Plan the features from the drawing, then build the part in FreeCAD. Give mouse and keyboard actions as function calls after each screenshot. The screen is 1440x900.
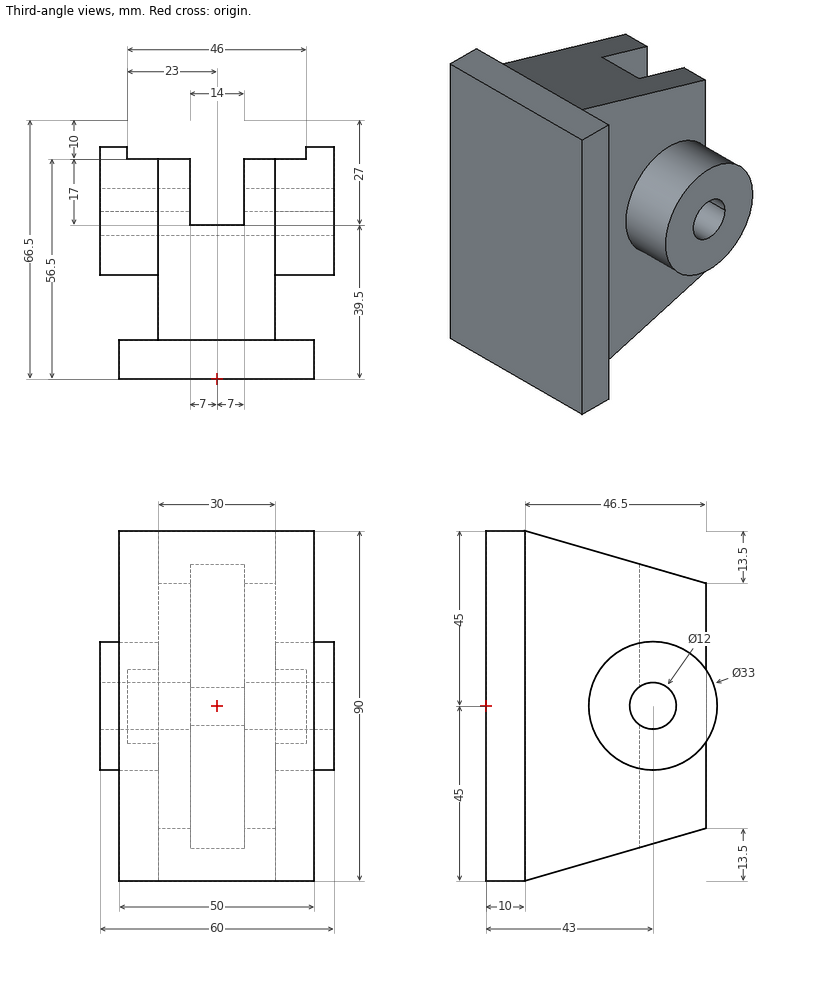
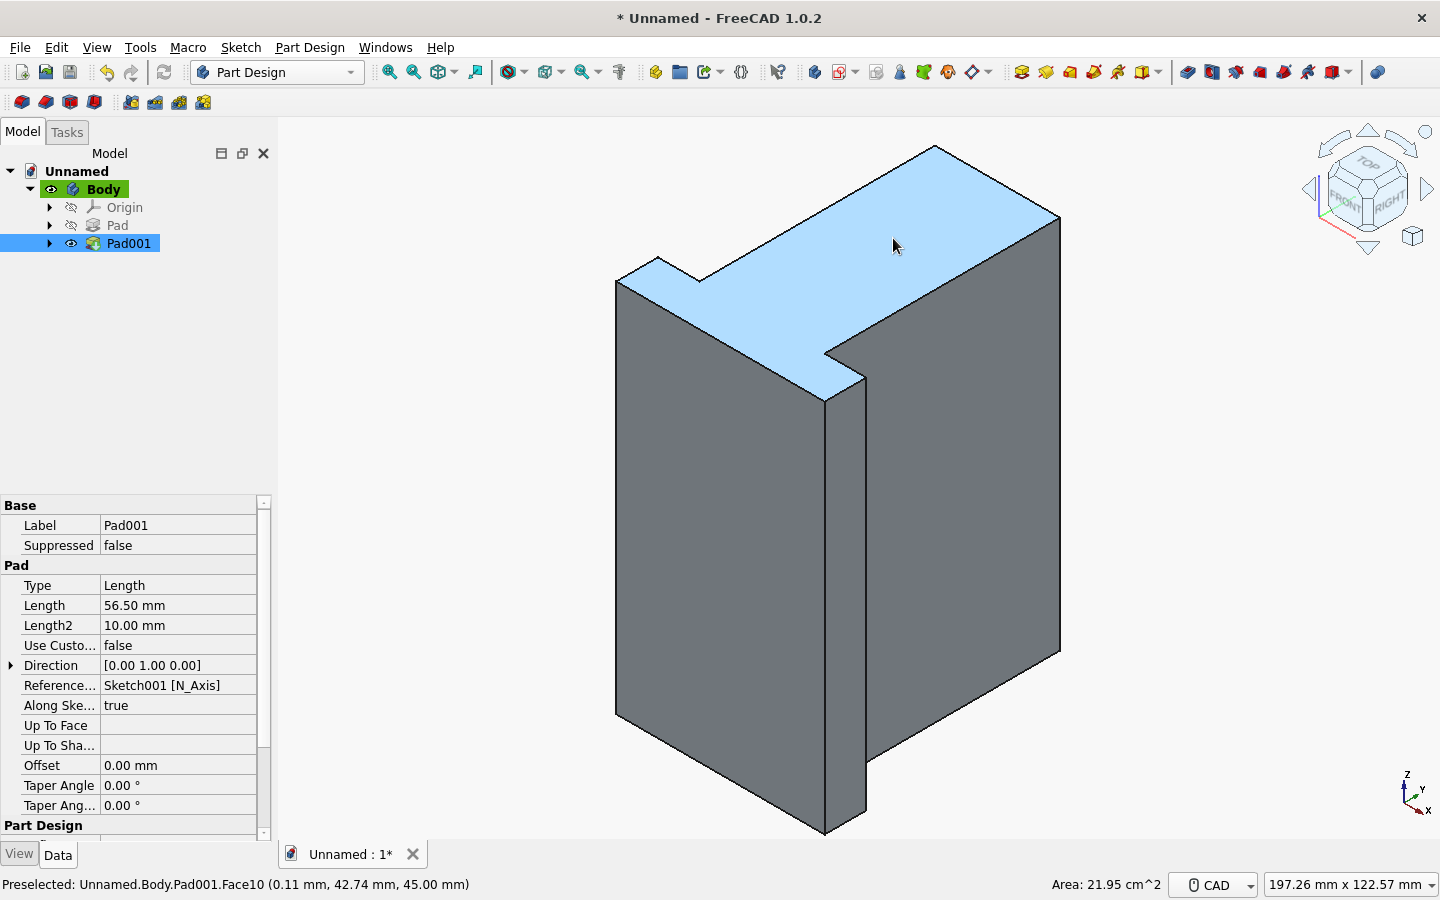
click(840, 72)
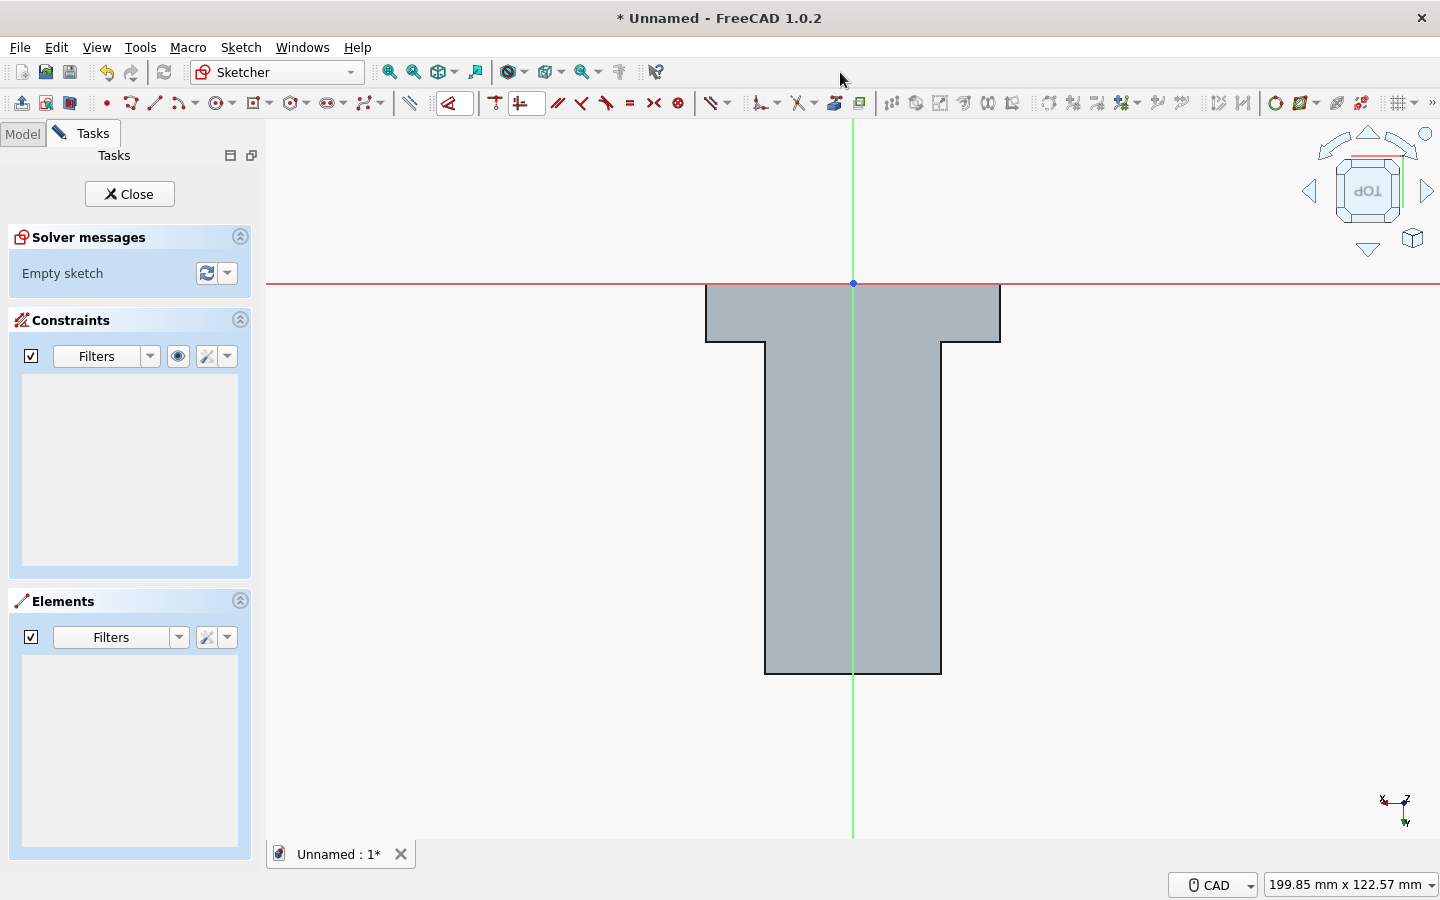
click(272, 104)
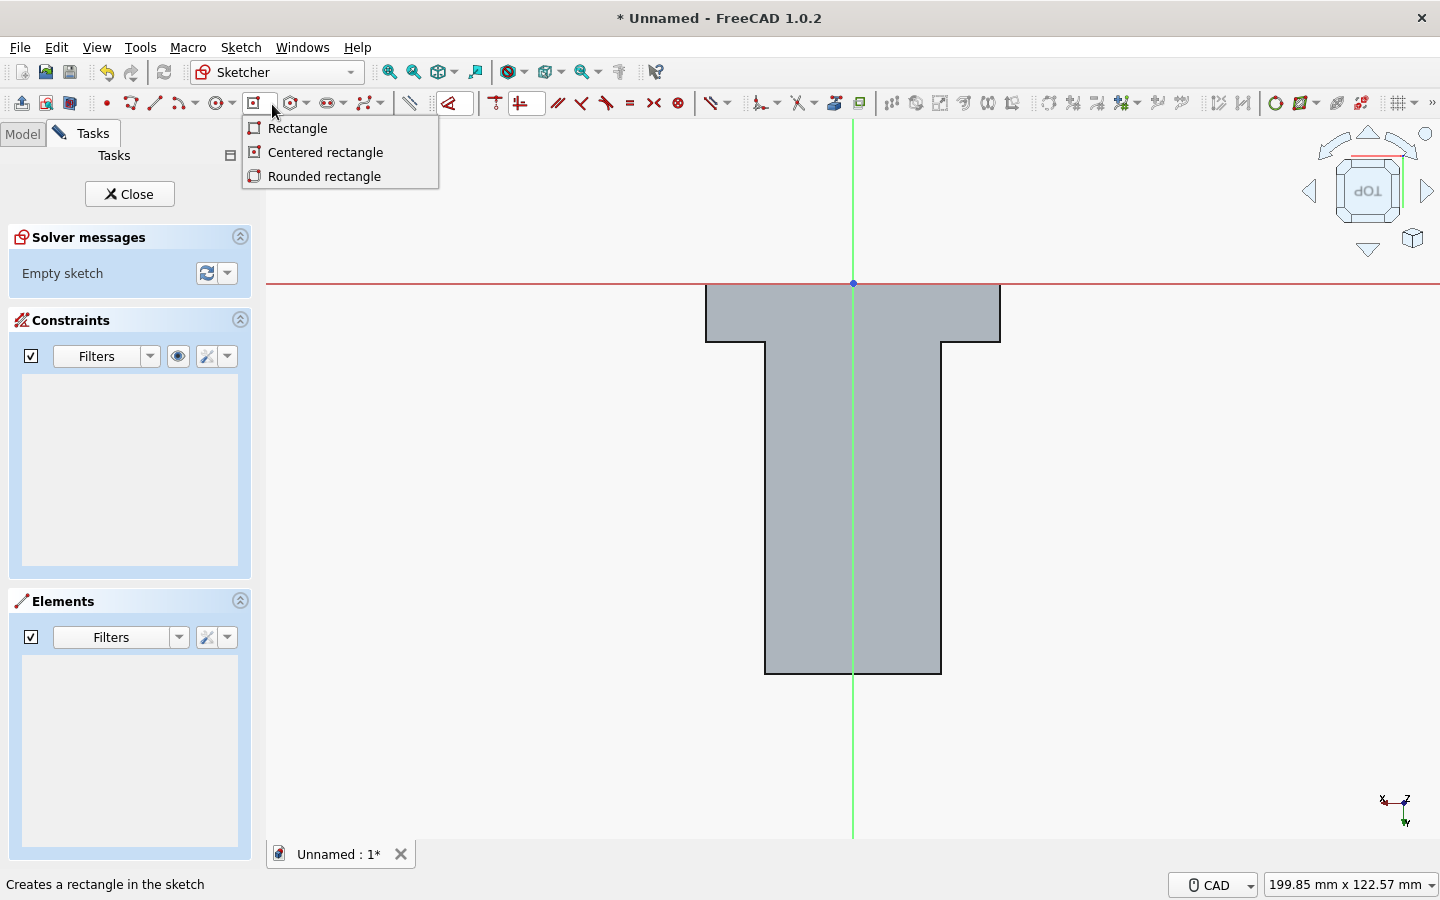
click(340, 128)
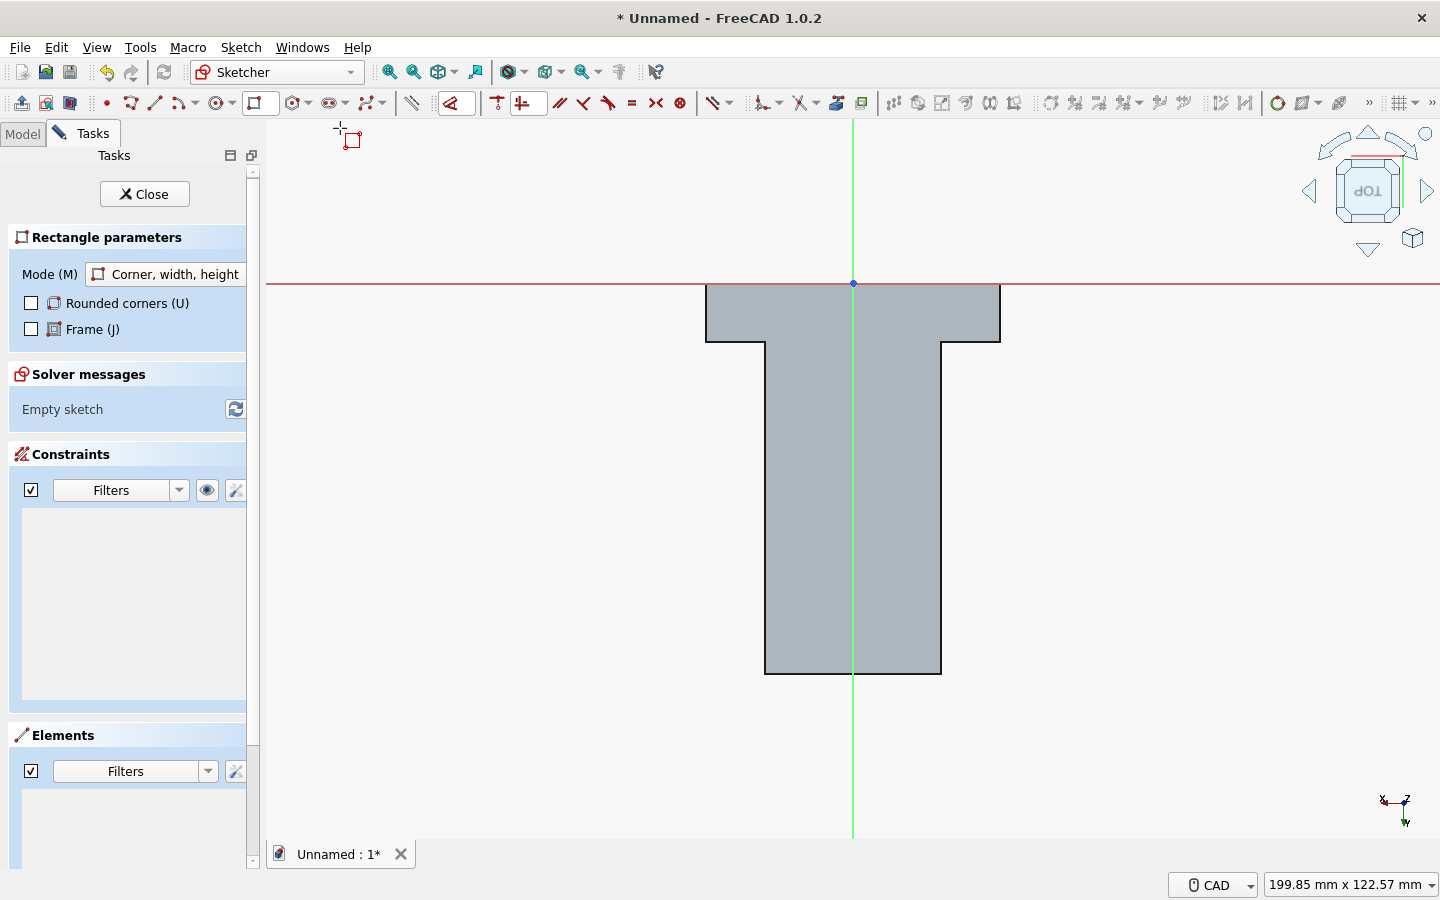
click(812, 516)
click(894, 674)
key(Escape)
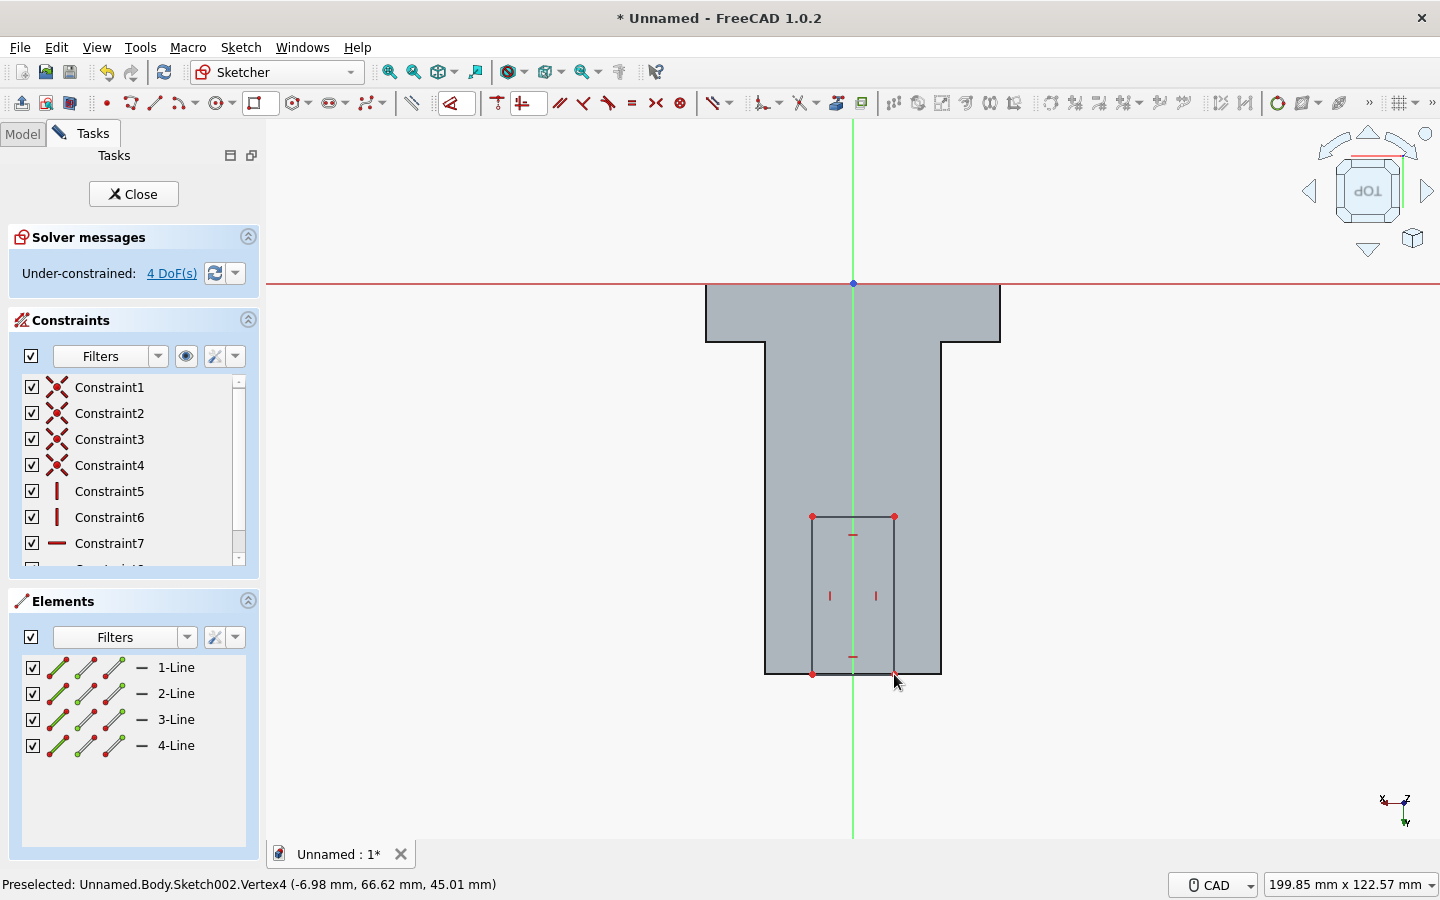
click(812, 564)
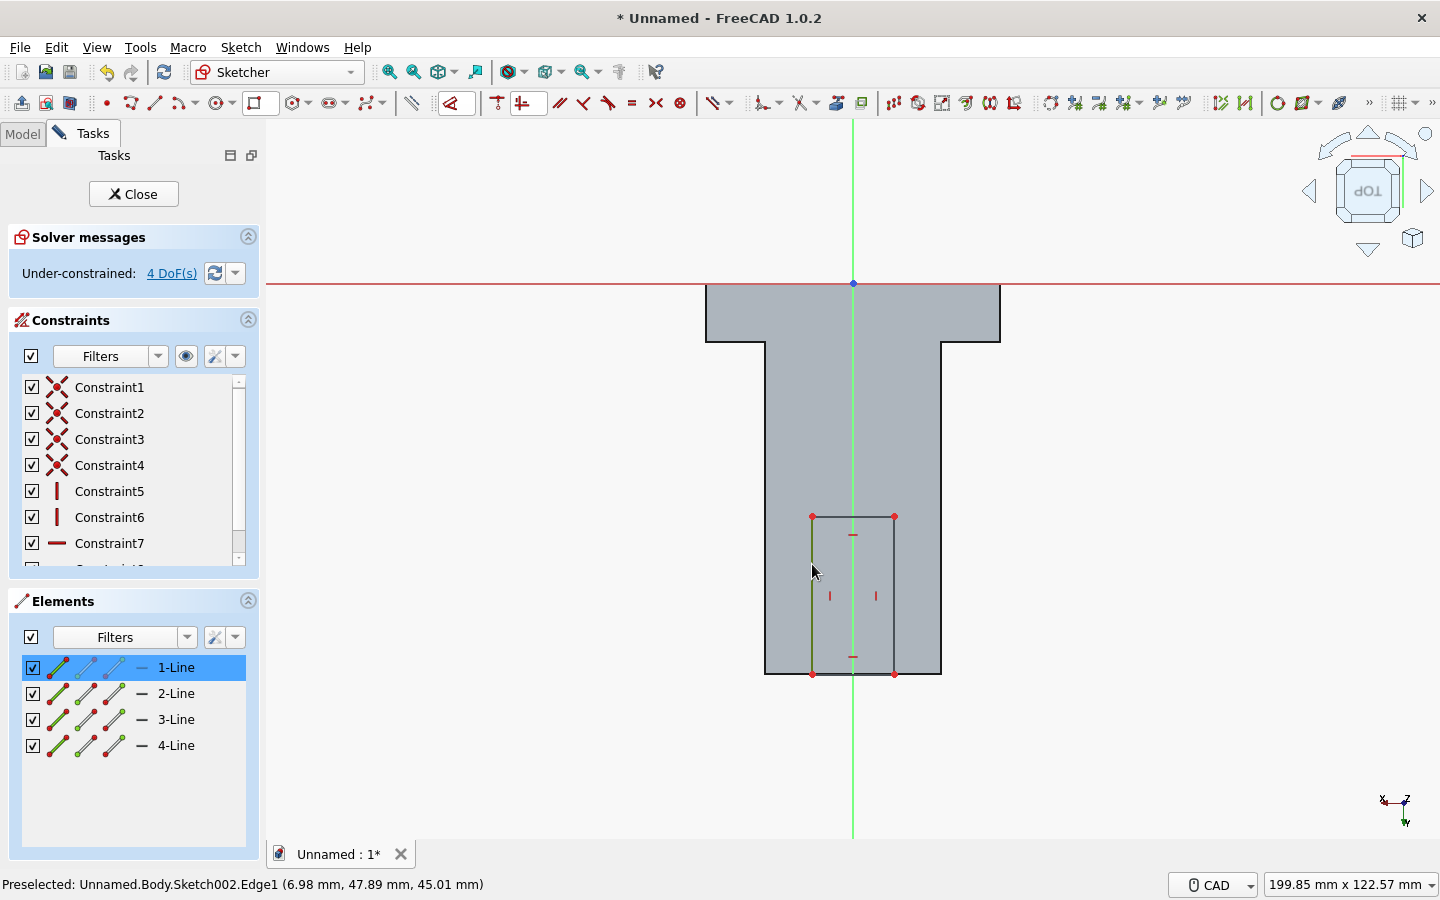
click(470, 104)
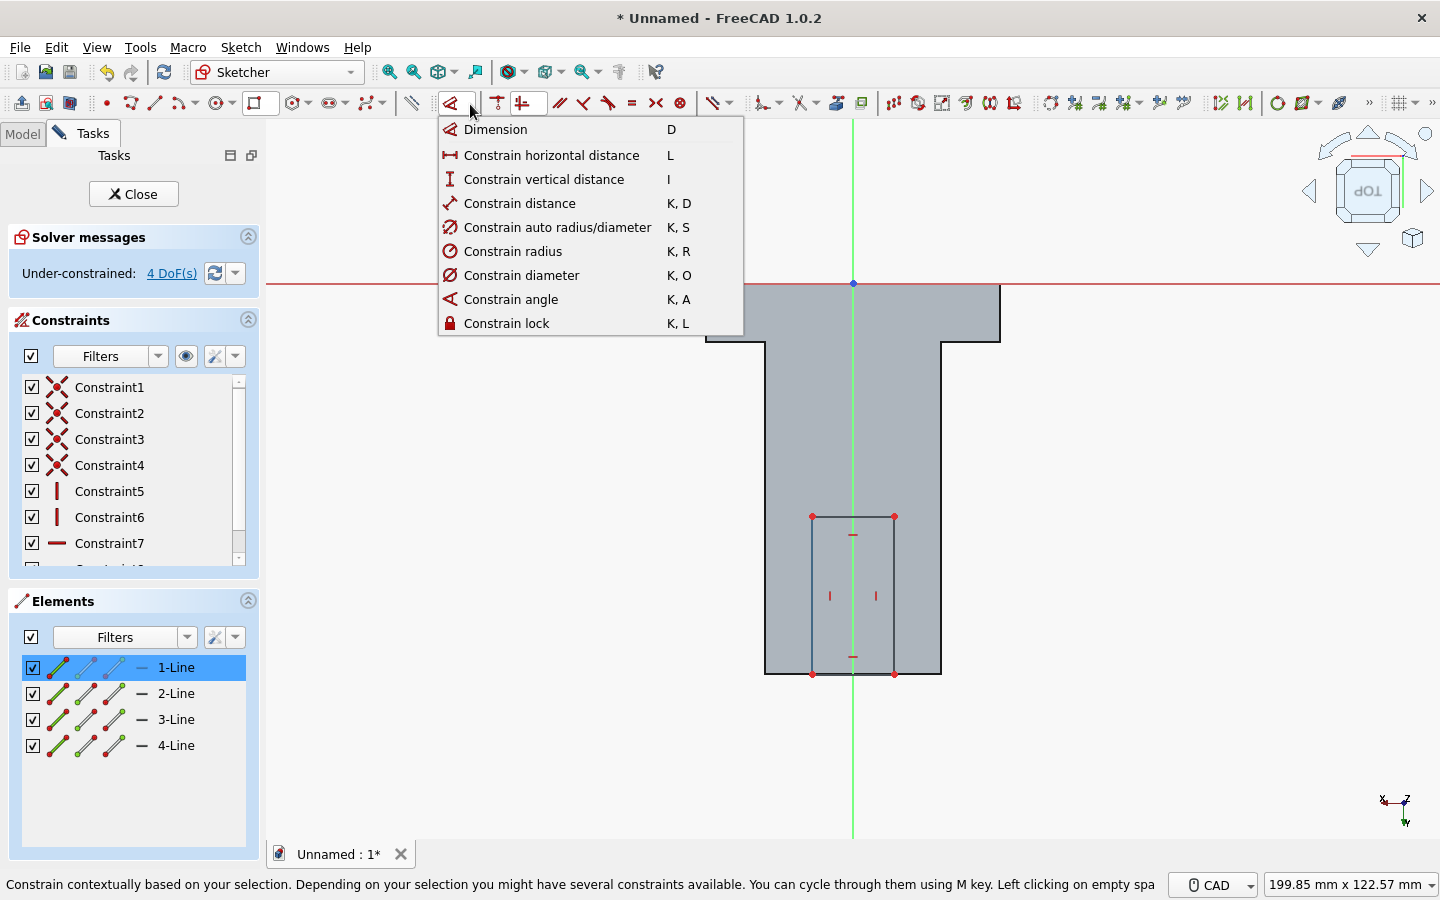
click(591, 179)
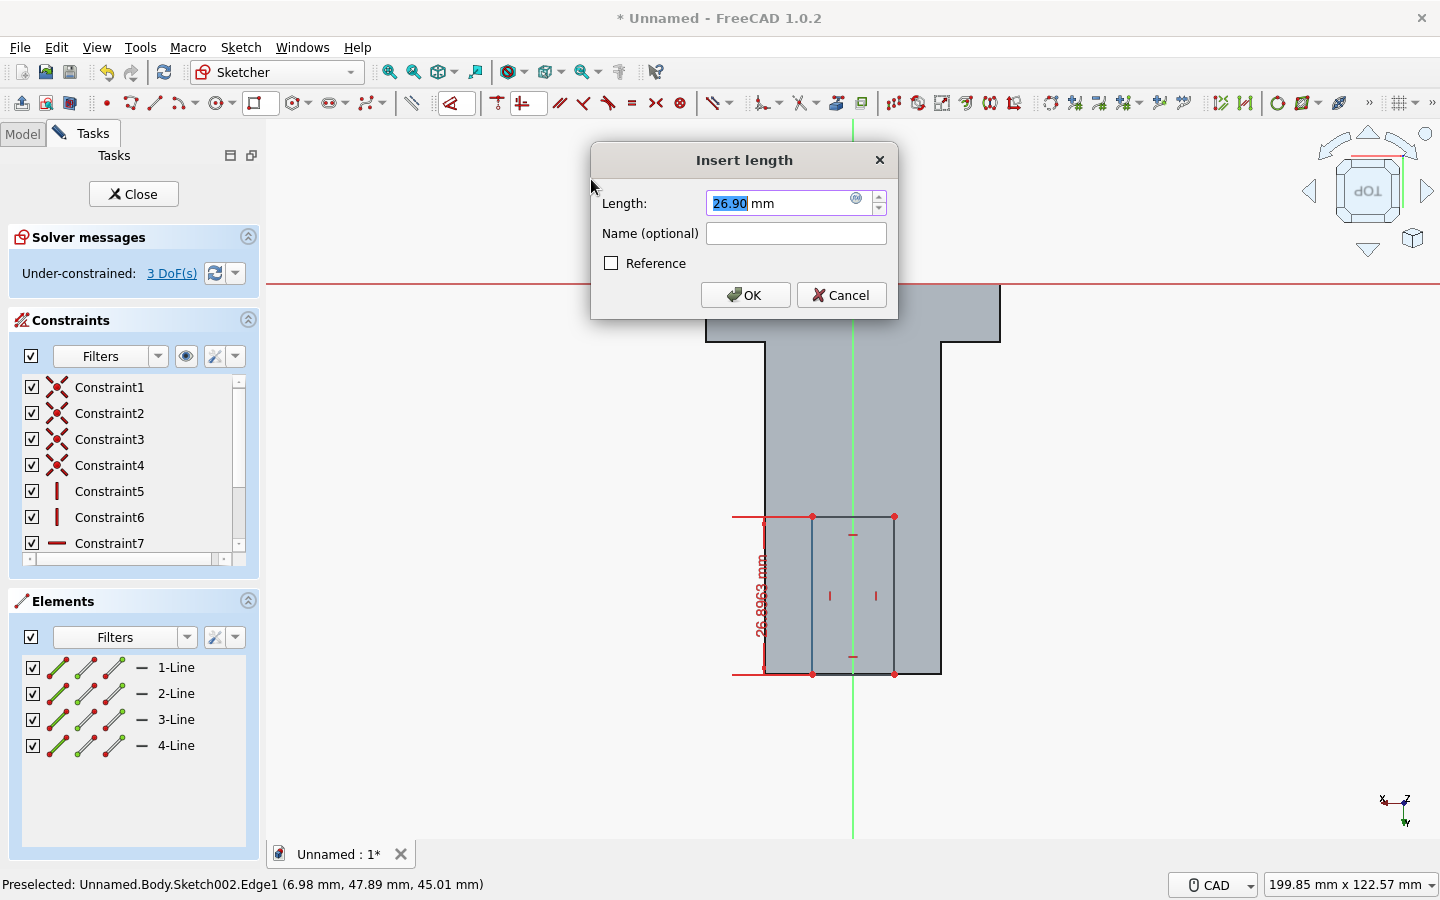
text(27)
key(Return)